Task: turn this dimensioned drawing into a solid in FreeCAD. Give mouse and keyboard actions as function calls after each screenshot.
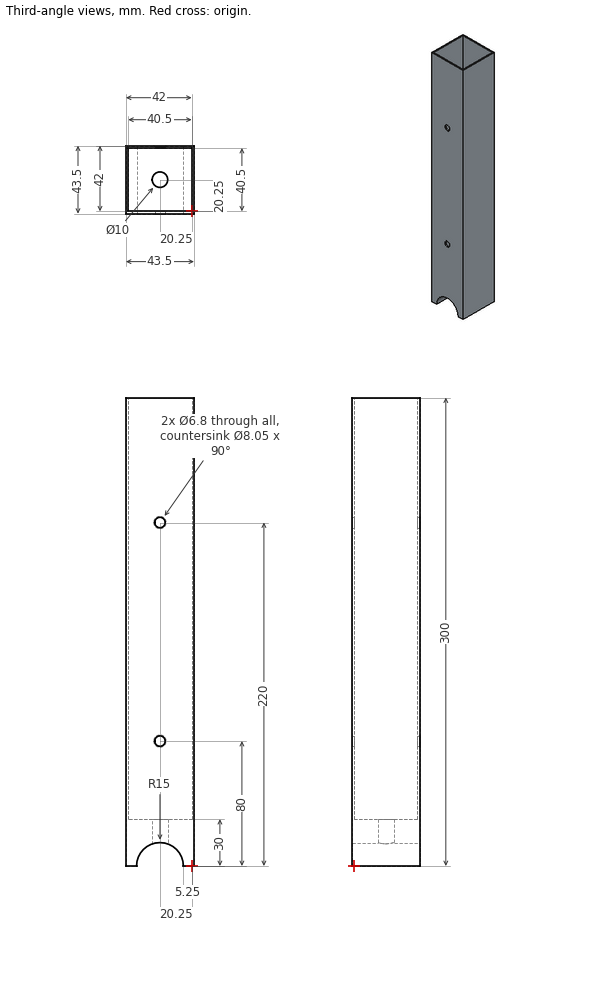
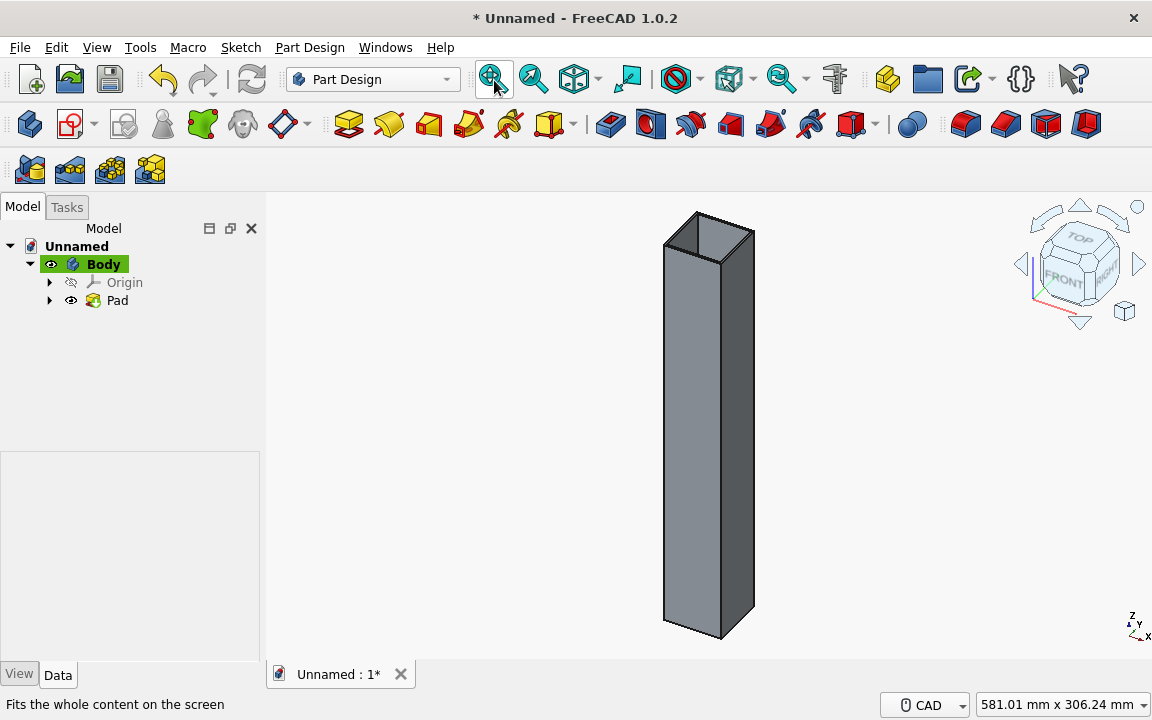
click(70, 124)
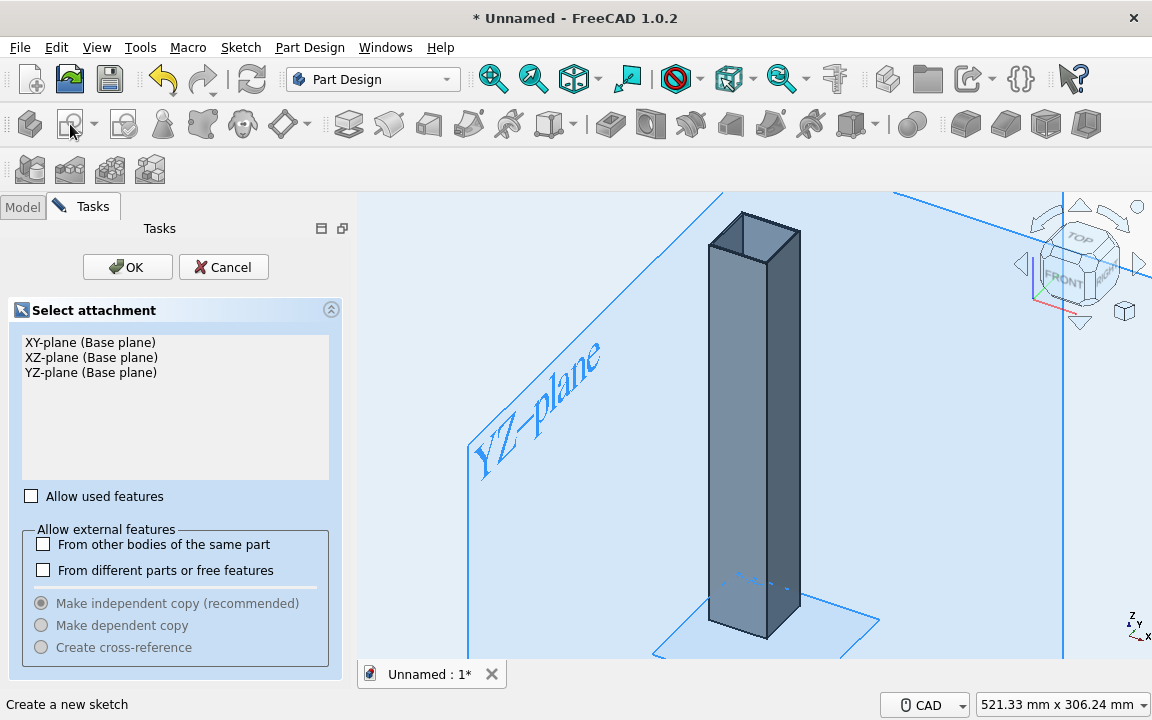
click(82, 342)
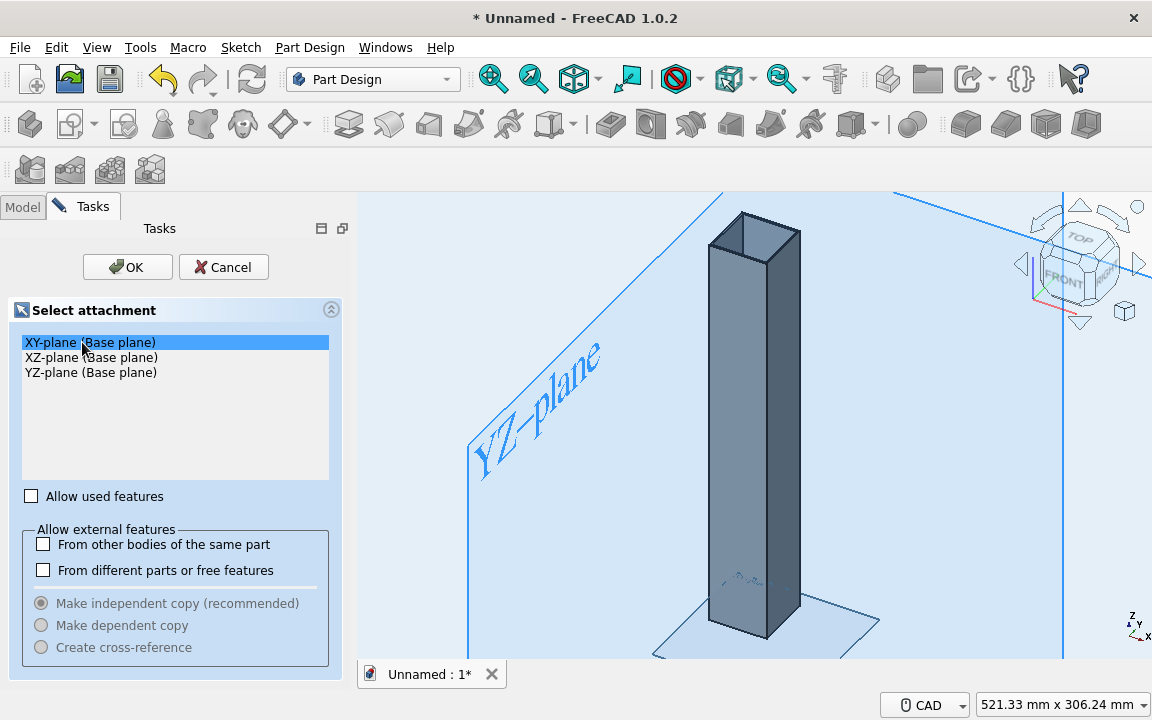
click(128, 267)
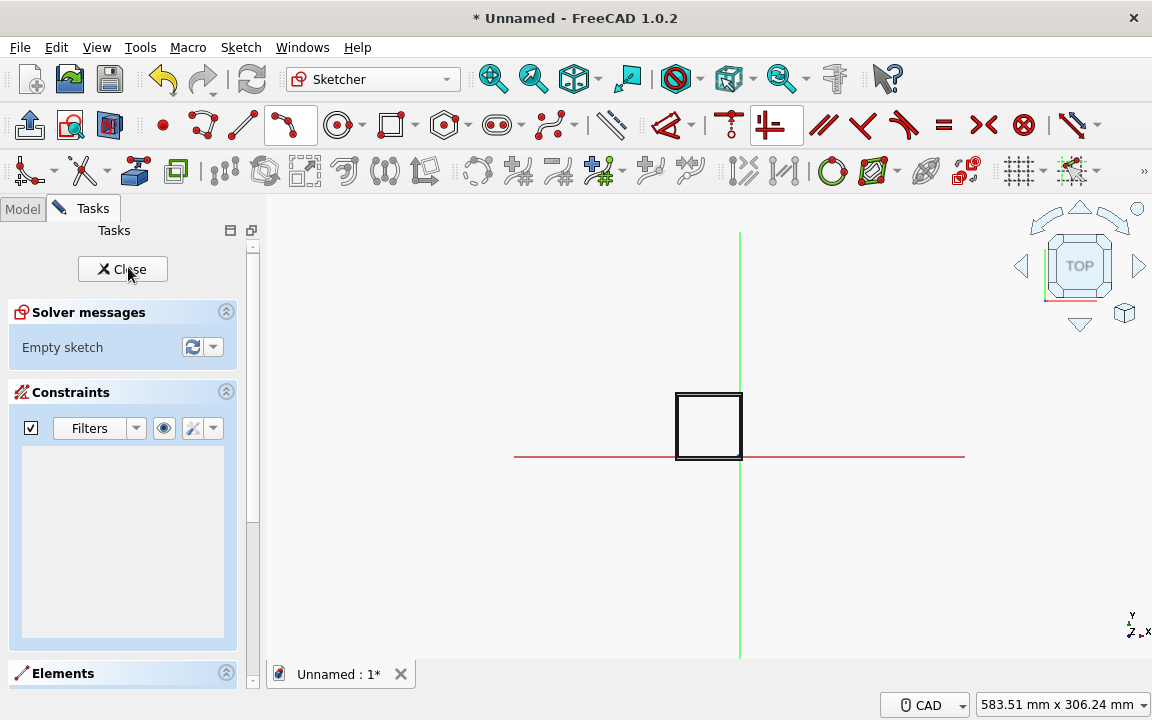
click(110, 126)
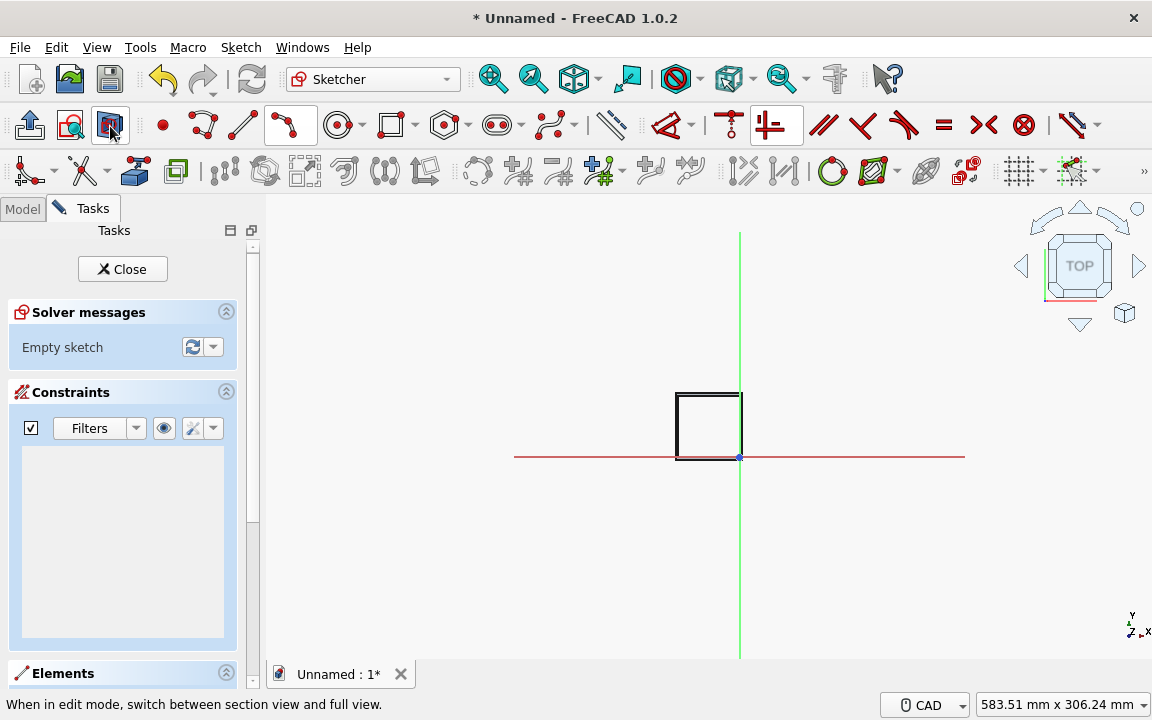
scroll(731, 426, up, 7)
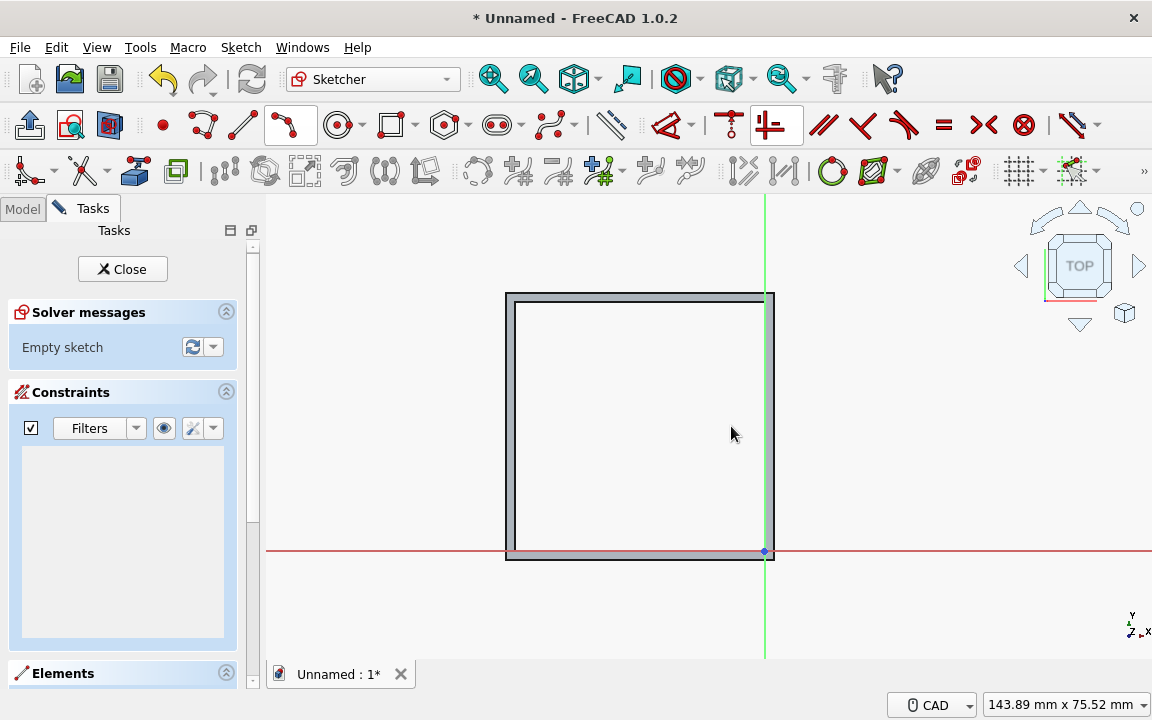
click(392, 126)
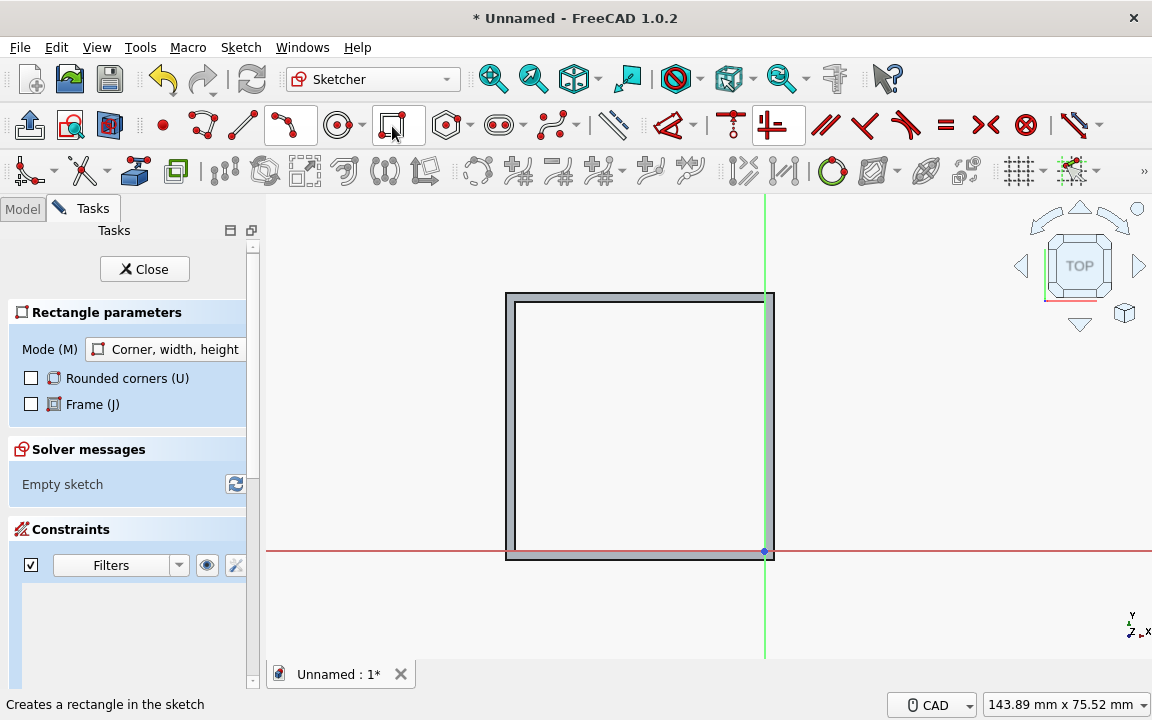
click(506, 293)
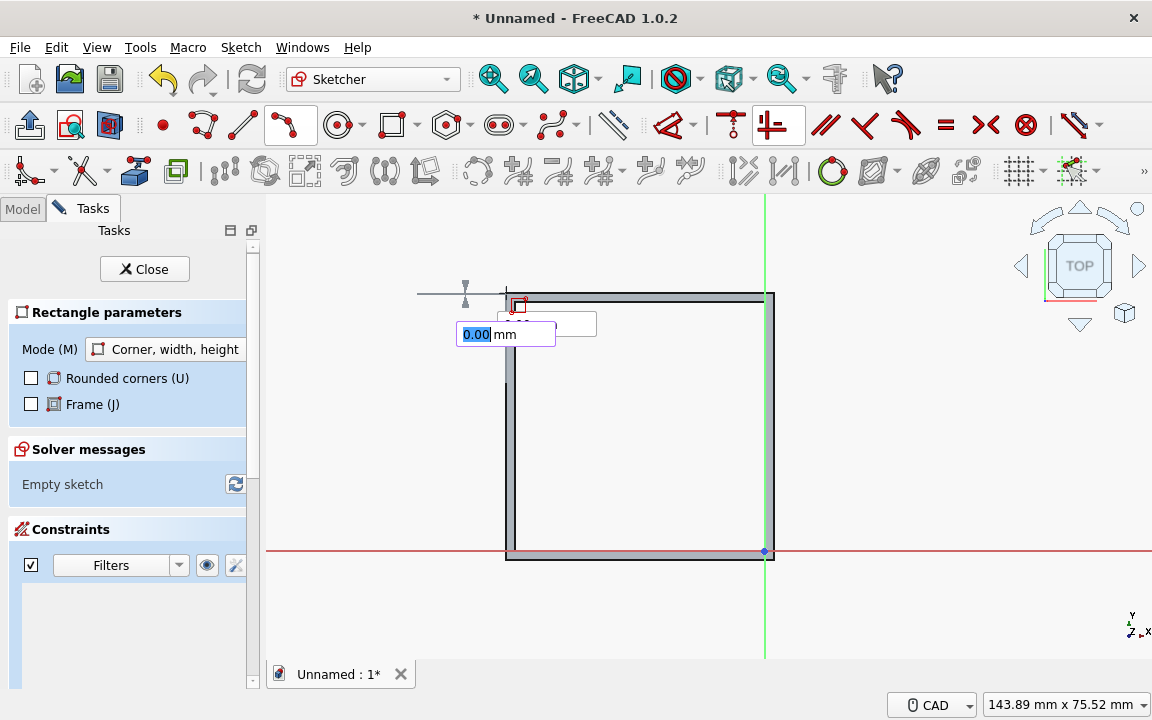
scroll(774, 560, up, 3)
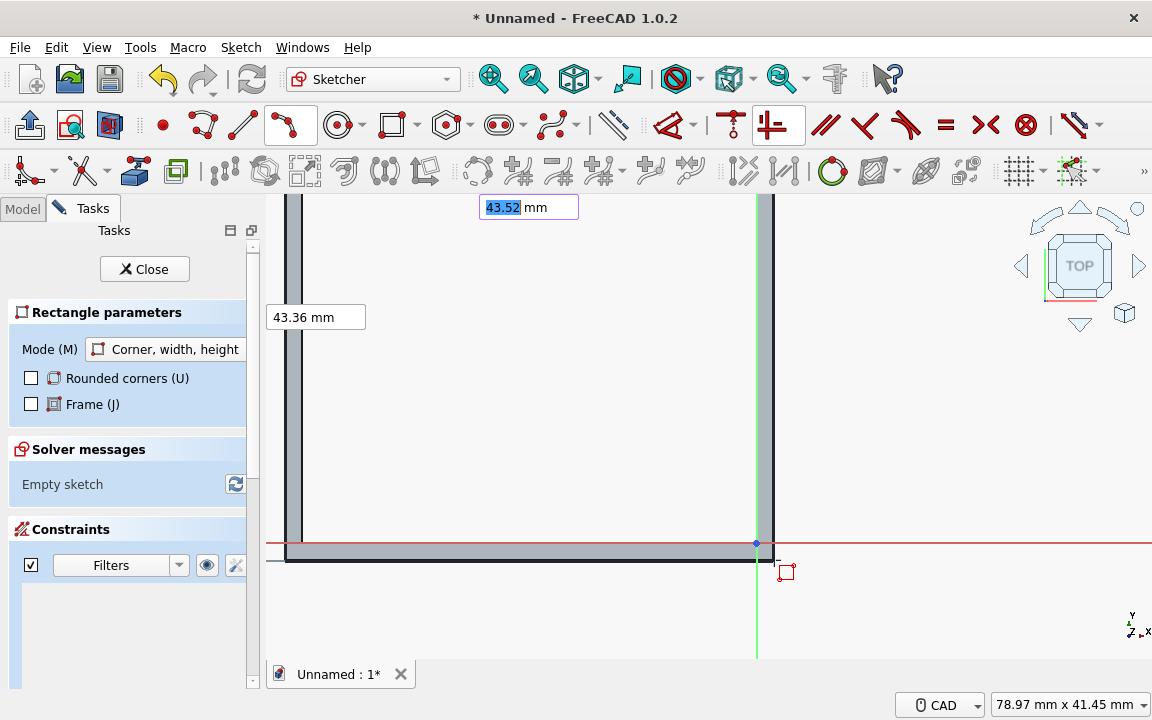
click(774, 560)
key(Escape)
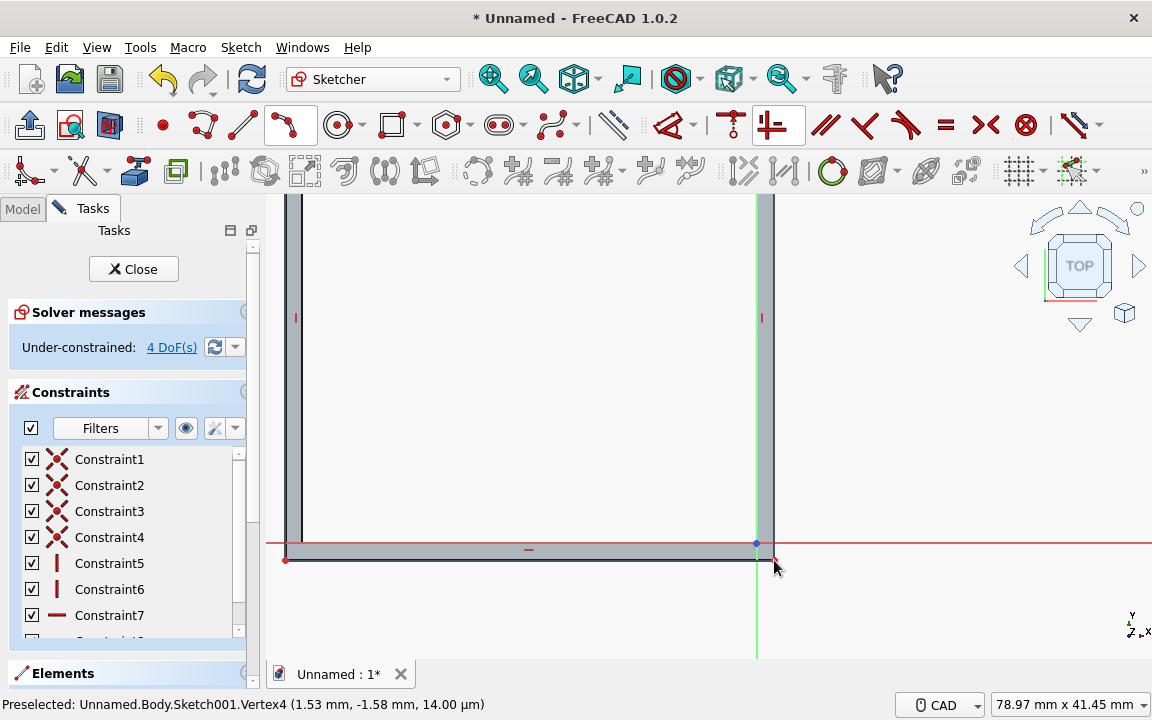
click(668, 126)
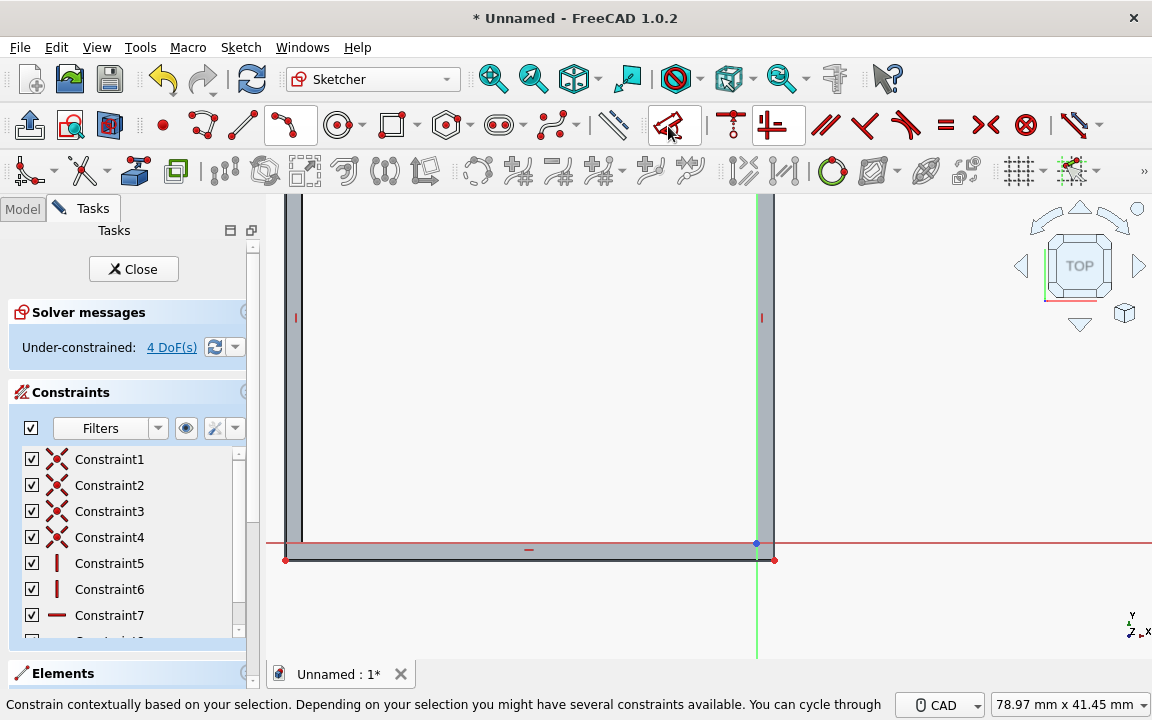
scroll(775, 561, down, 3)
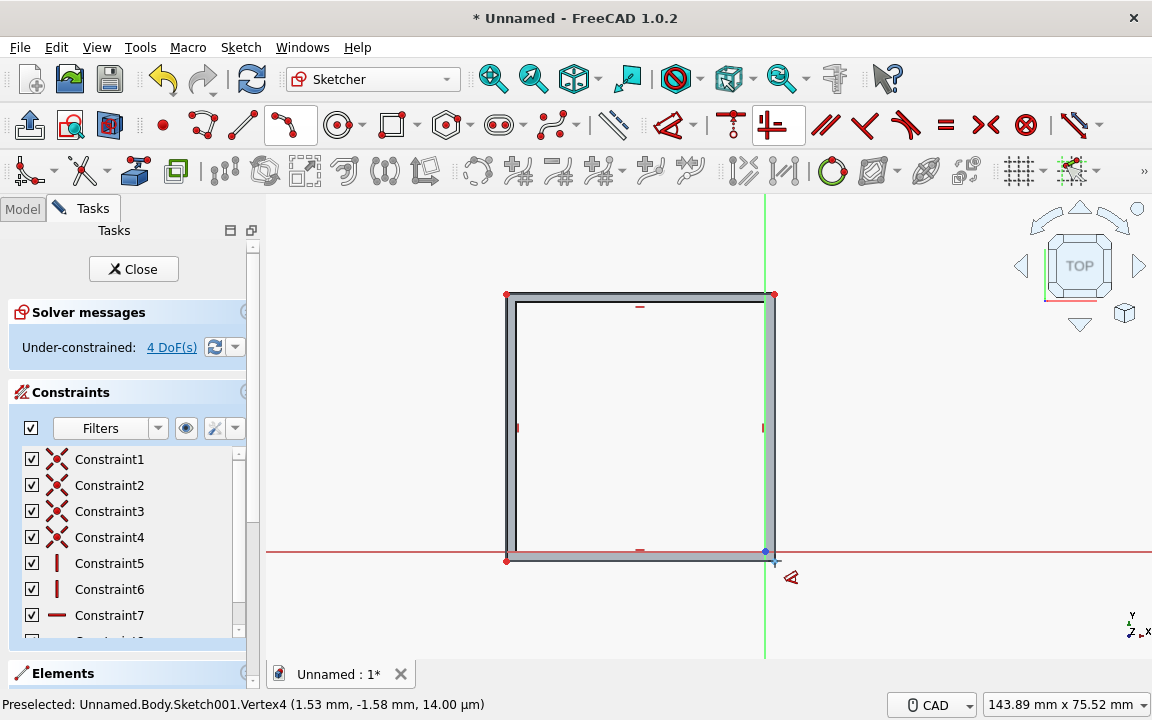
click(506, 294)
click(636, 260)